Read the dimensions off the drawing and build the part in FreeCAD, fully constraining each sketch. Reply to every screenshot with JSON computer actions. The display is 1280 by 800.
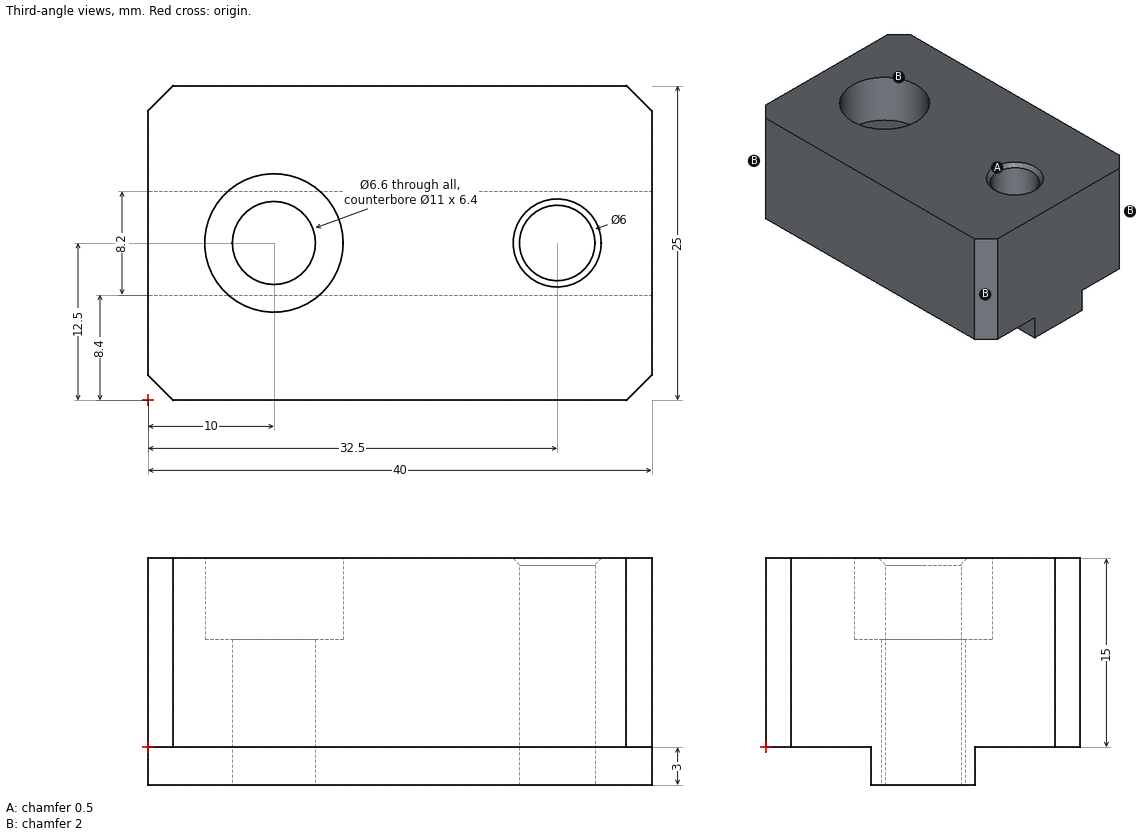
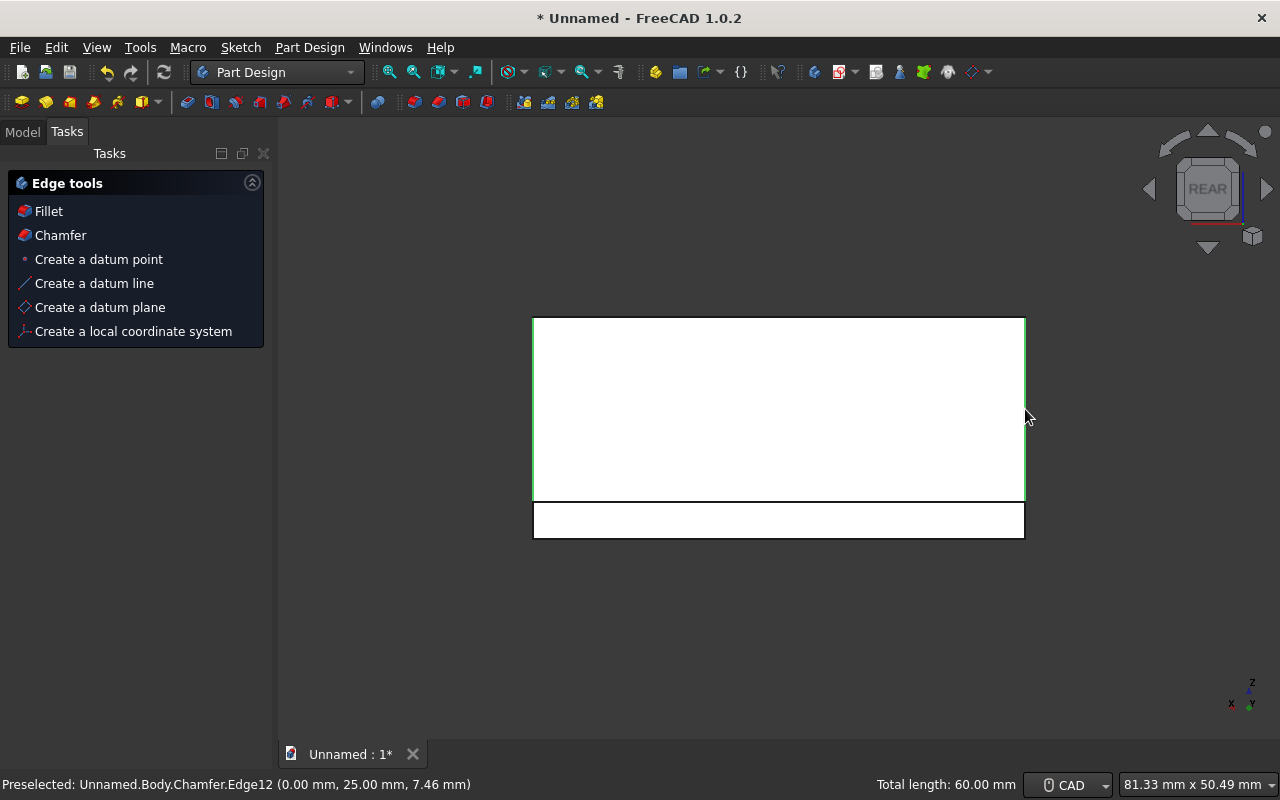
{"action": "left_click", "coordinate": [440, 102]}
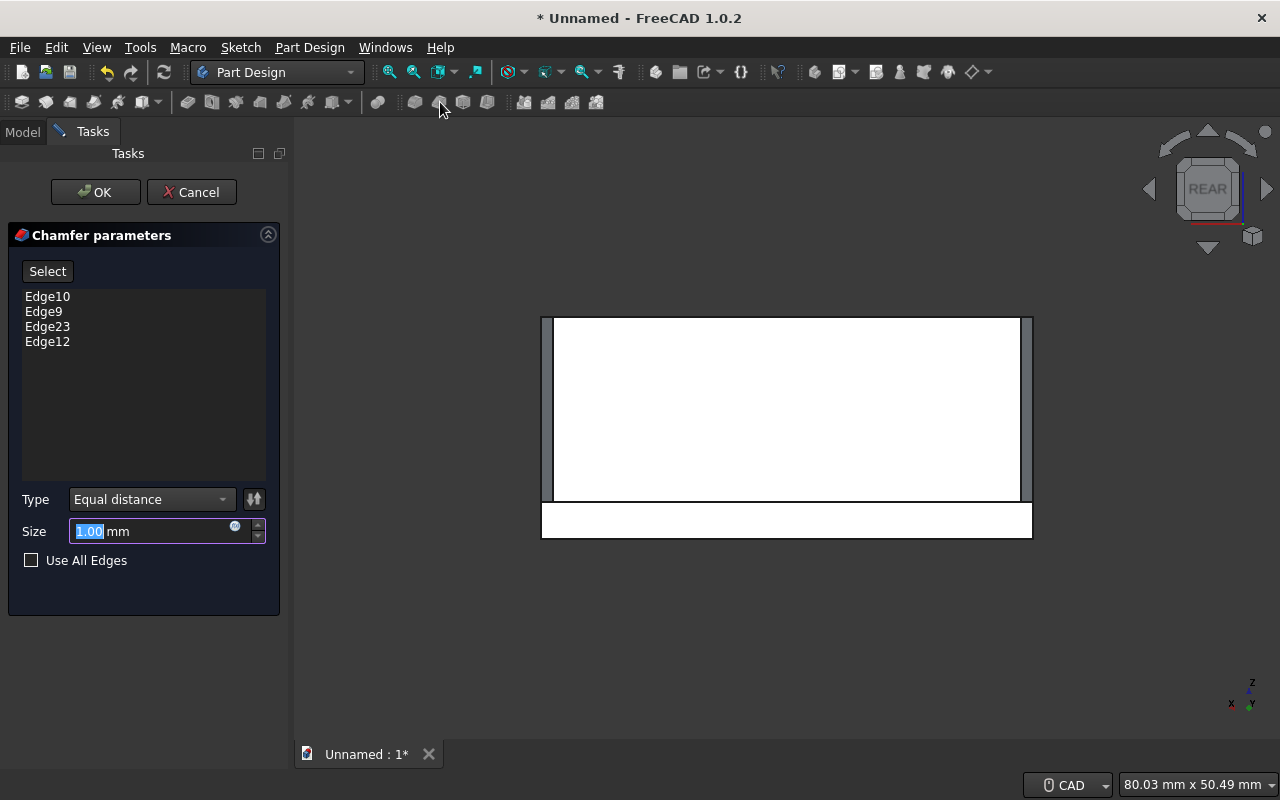
{"action": "type", "text": "2"}
{"action": "key", "text": "Tab"}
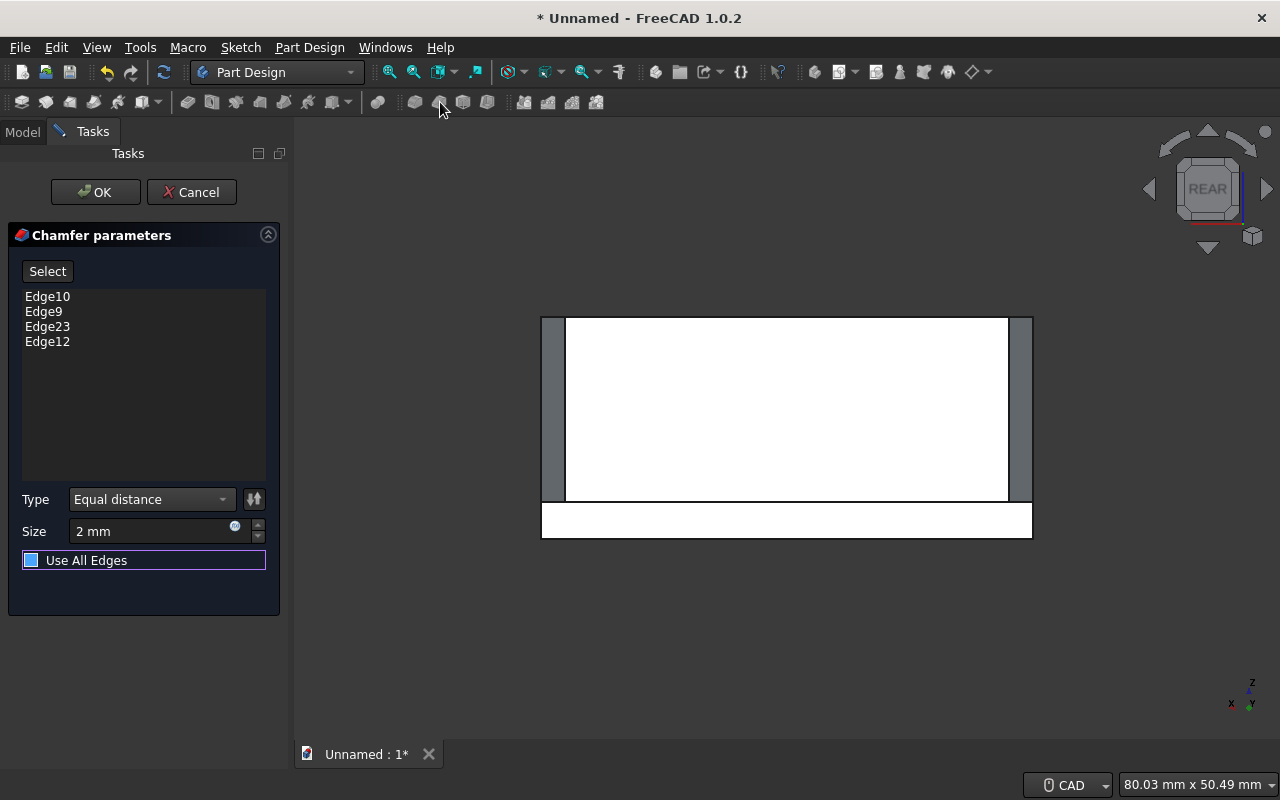
{"action": "left_click", "coordinate": [96, 192]}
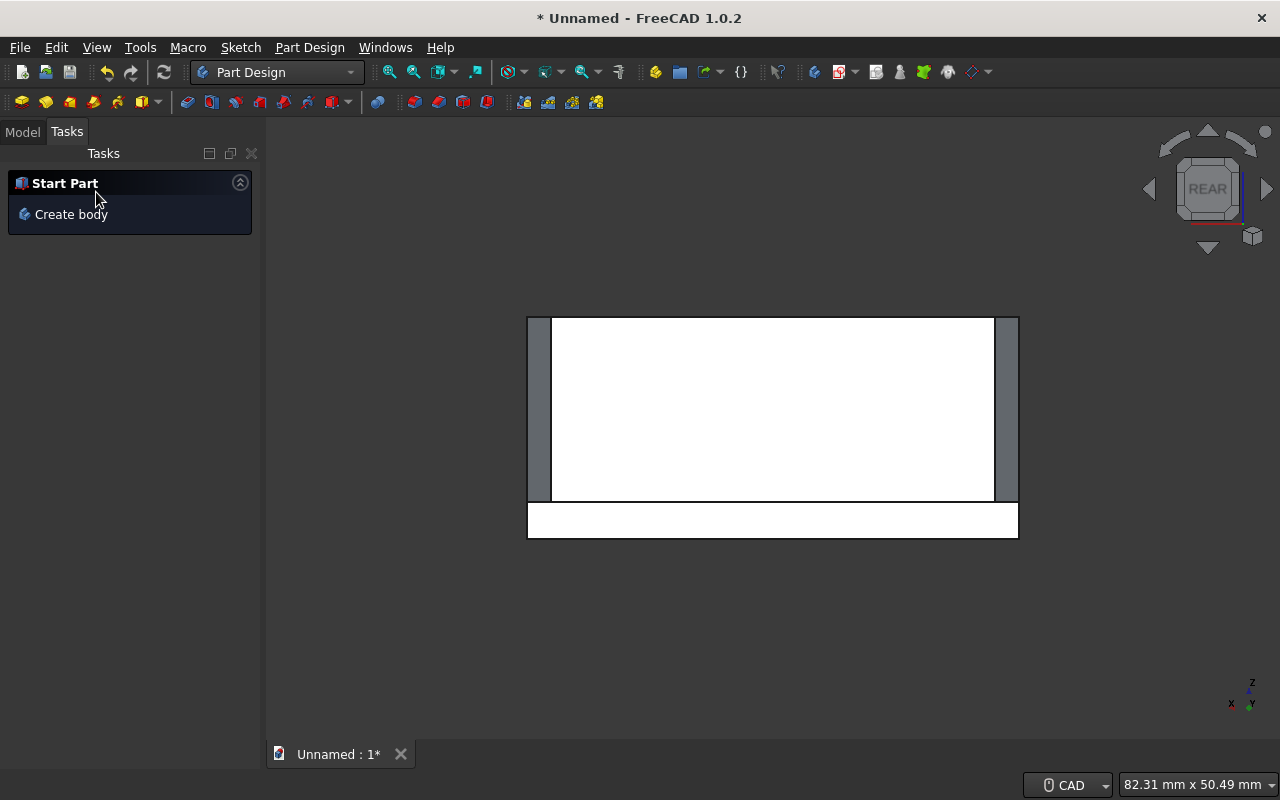
{"action": "key", "text": "0"}